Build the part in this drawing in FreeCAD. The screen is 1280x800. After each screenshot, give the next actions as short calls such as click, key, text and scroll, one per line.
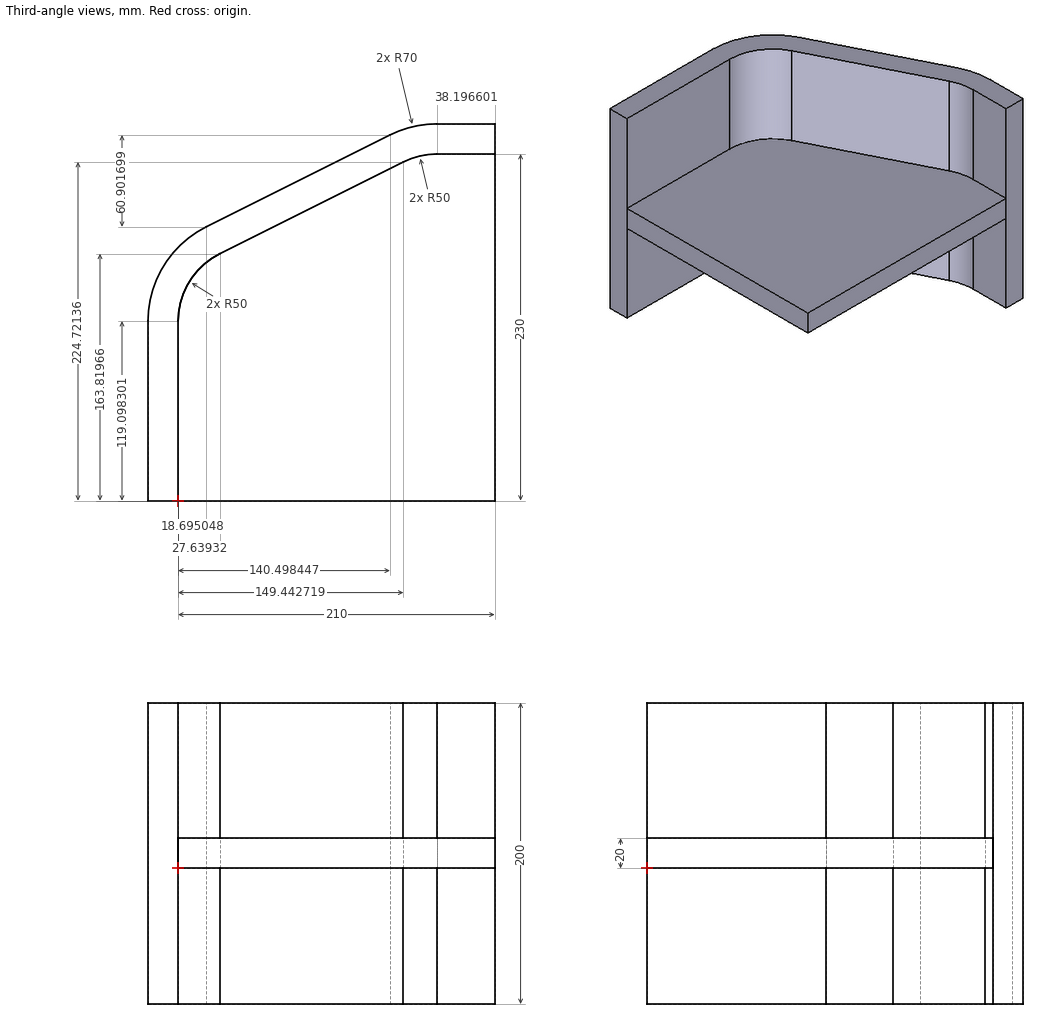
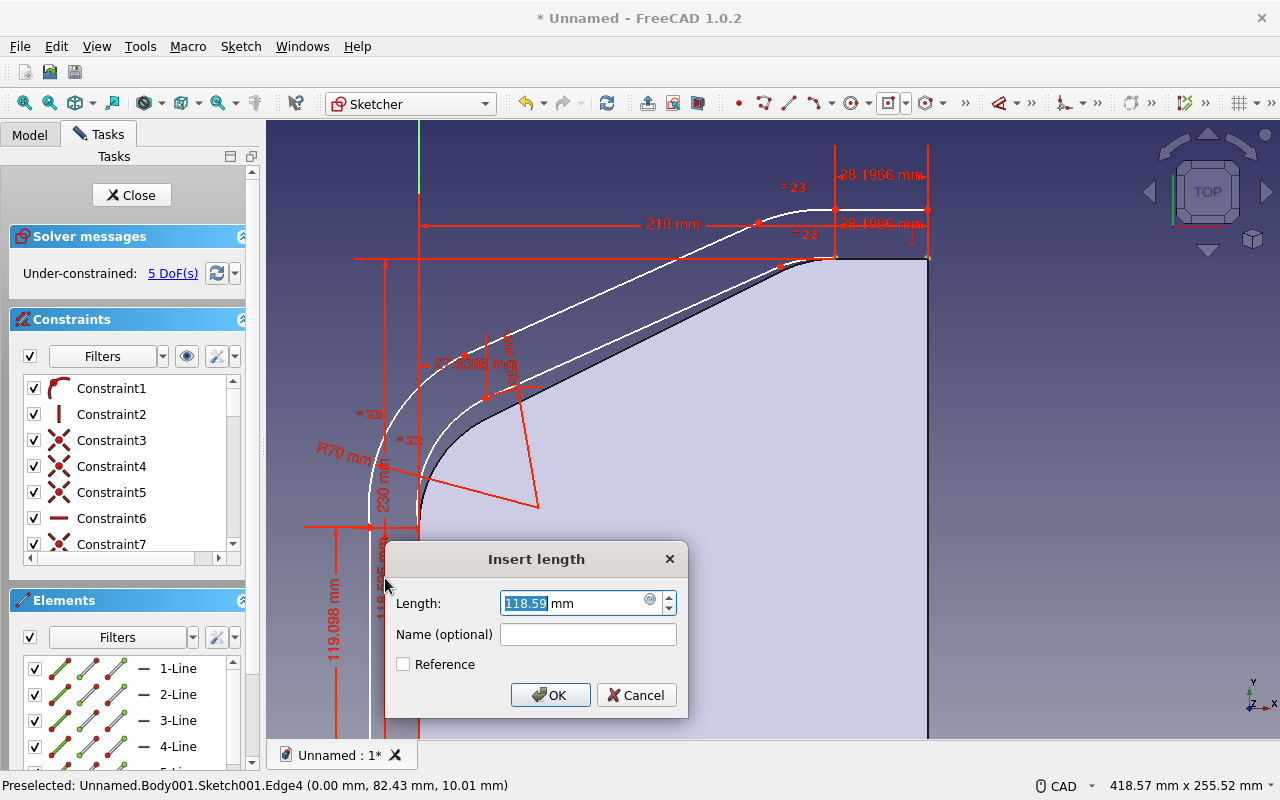
text(119.098301)
key(Return)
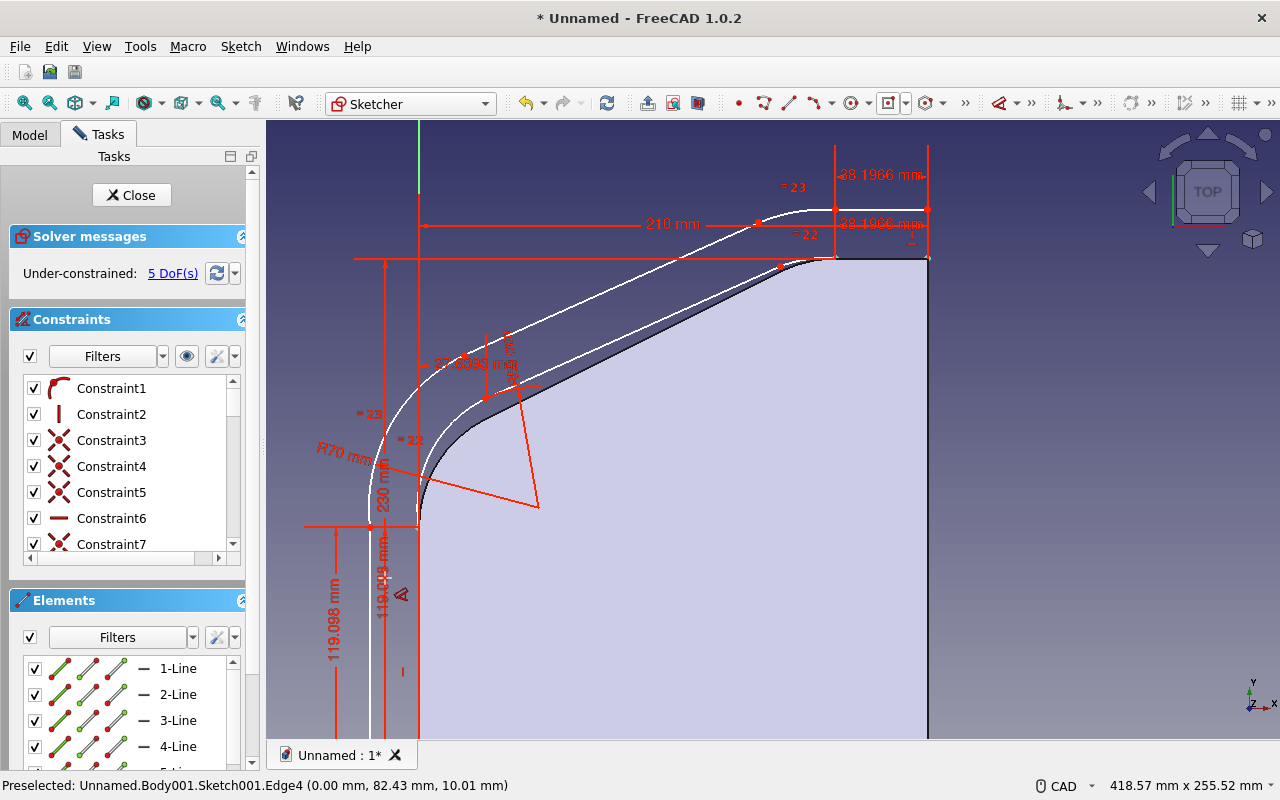
click(465, 355)
click(442, 321)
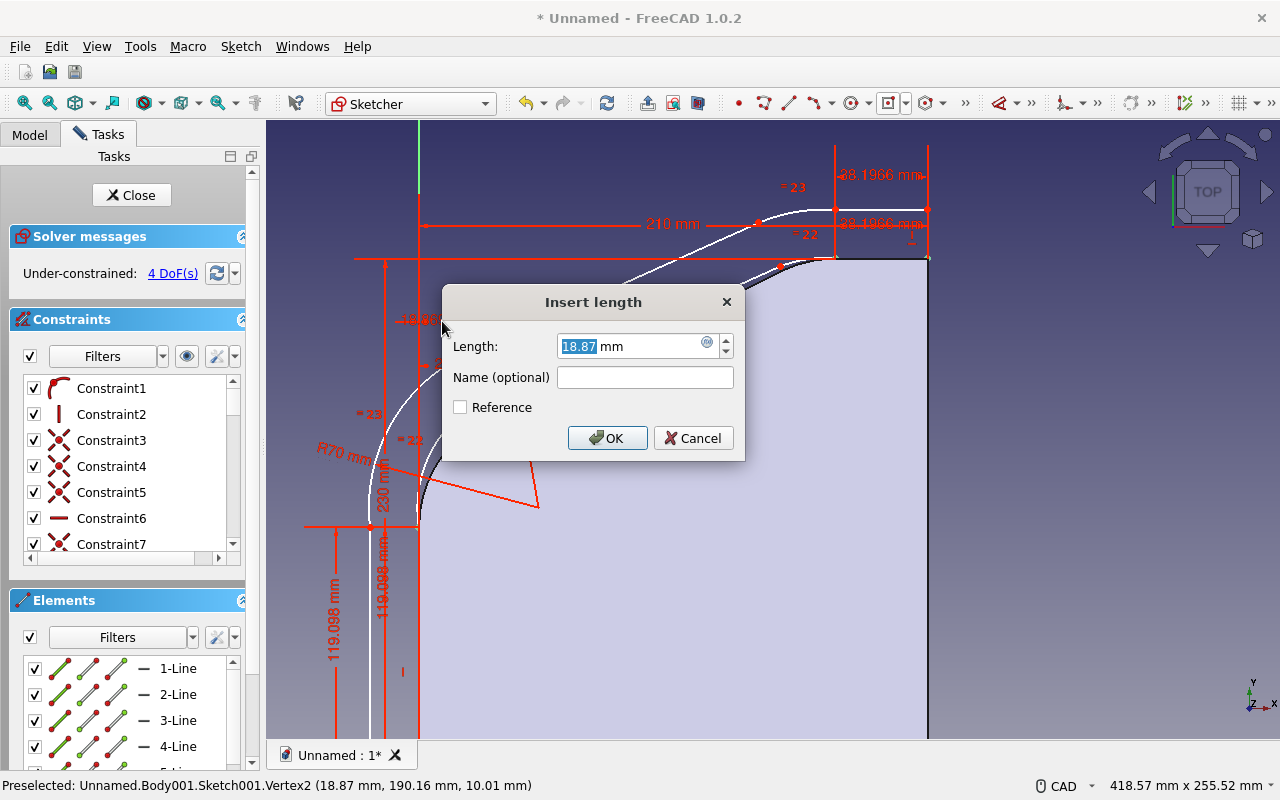
text(18.695048)
key(Return)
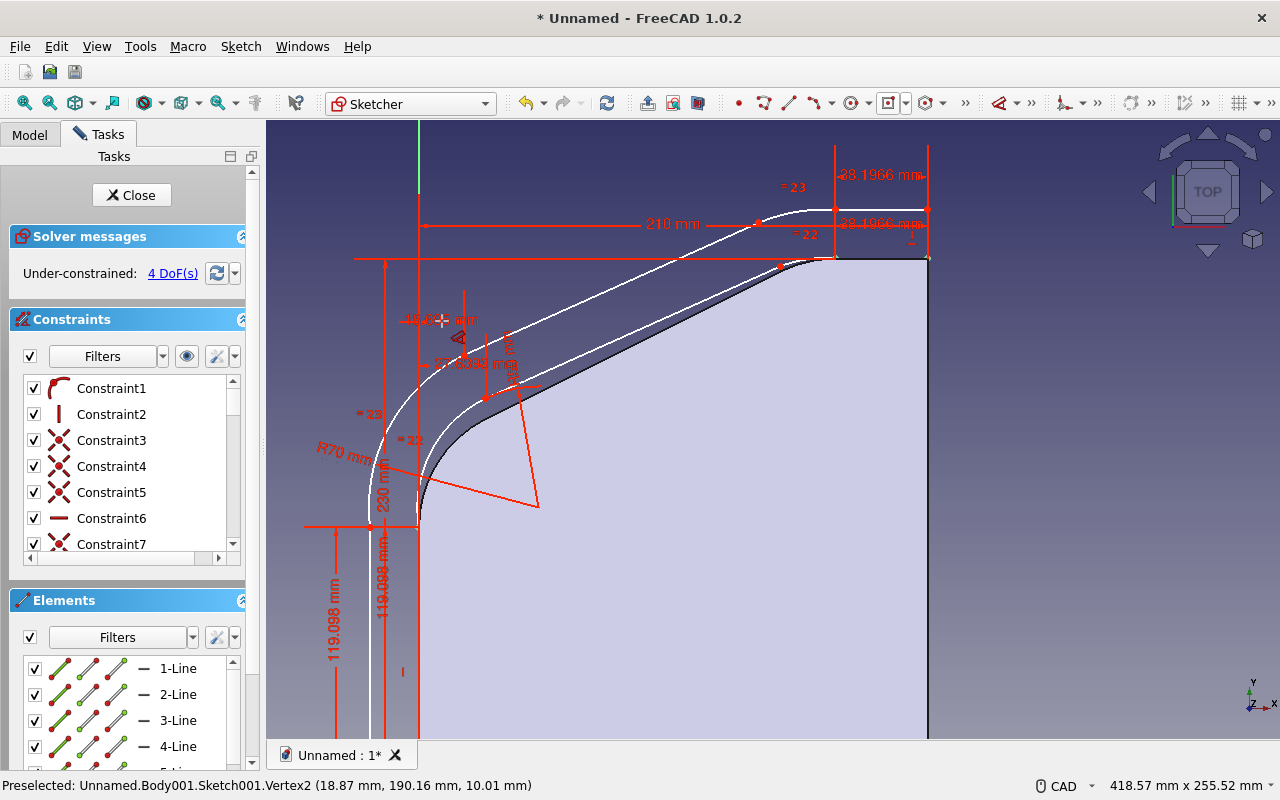
click(486, 398)
click(385, 555)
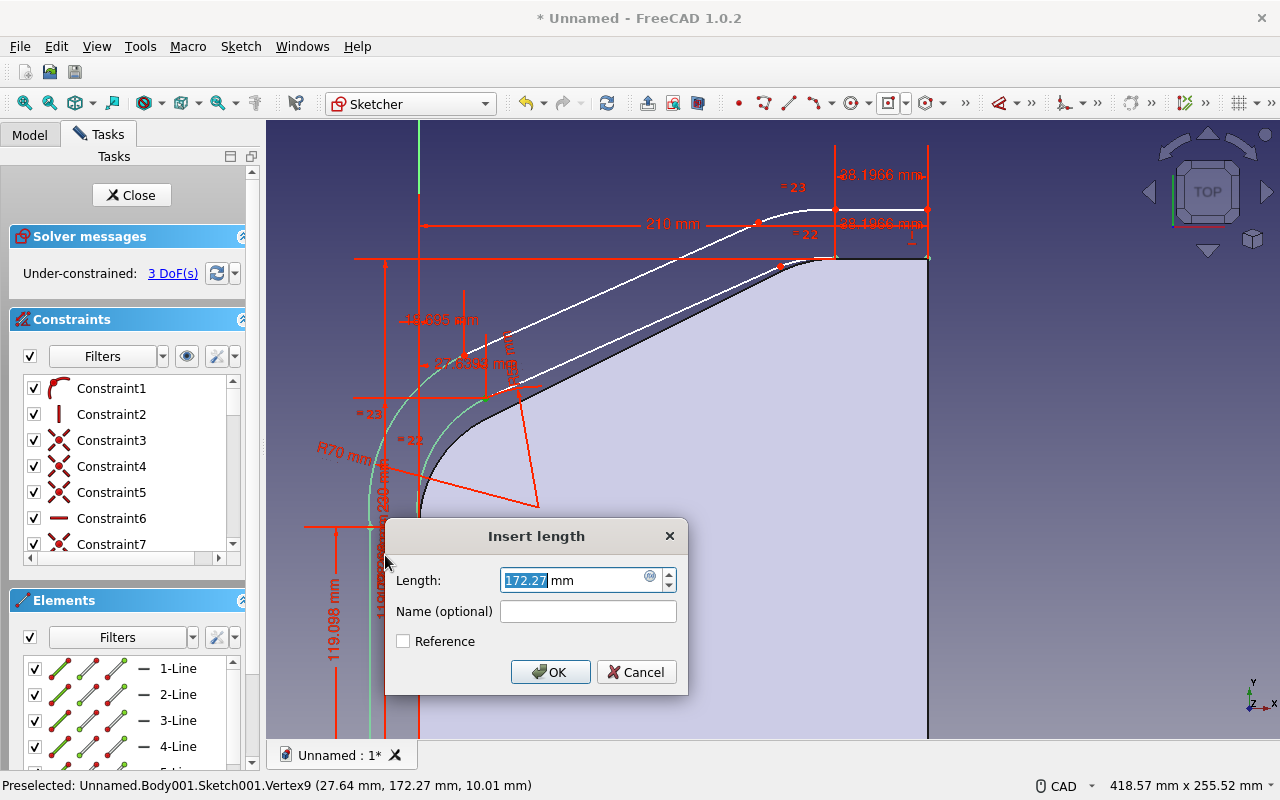
text(163.81966)
key(Return)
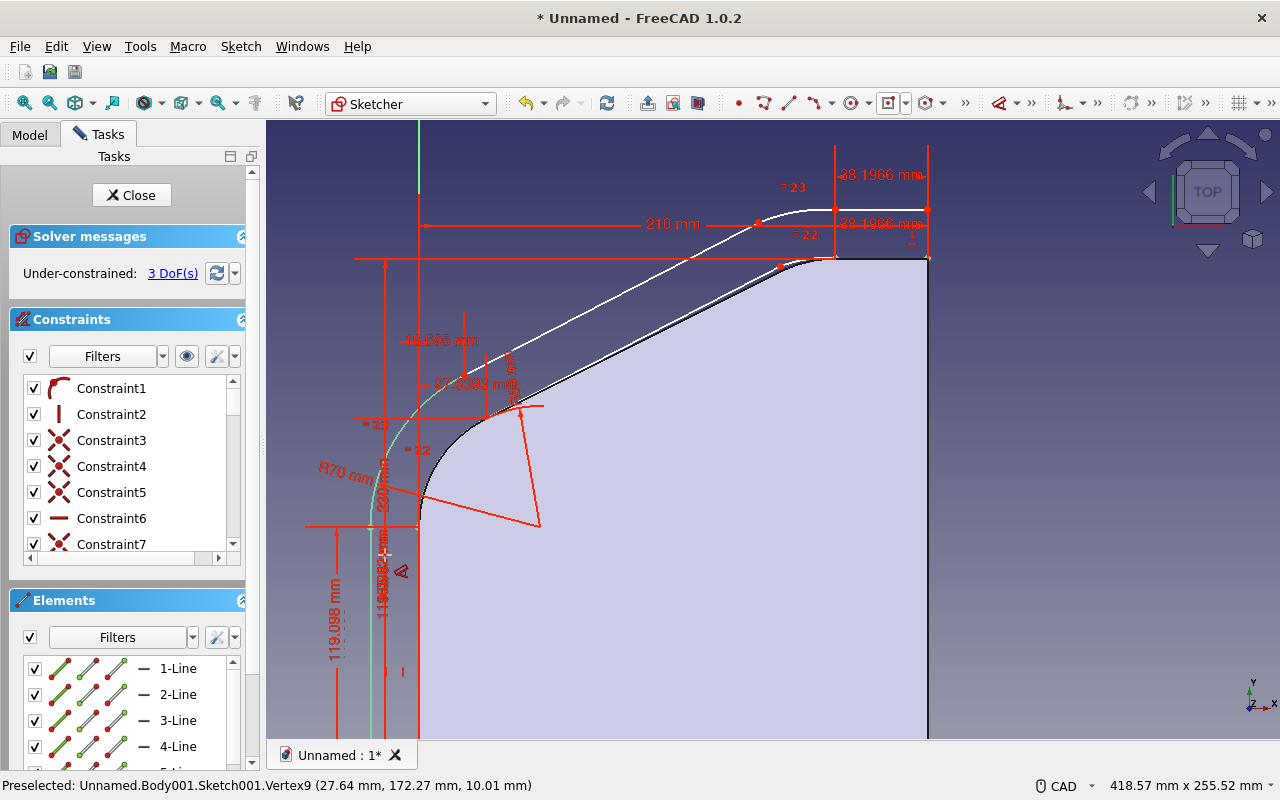
click(781, 266)
click(385, 386)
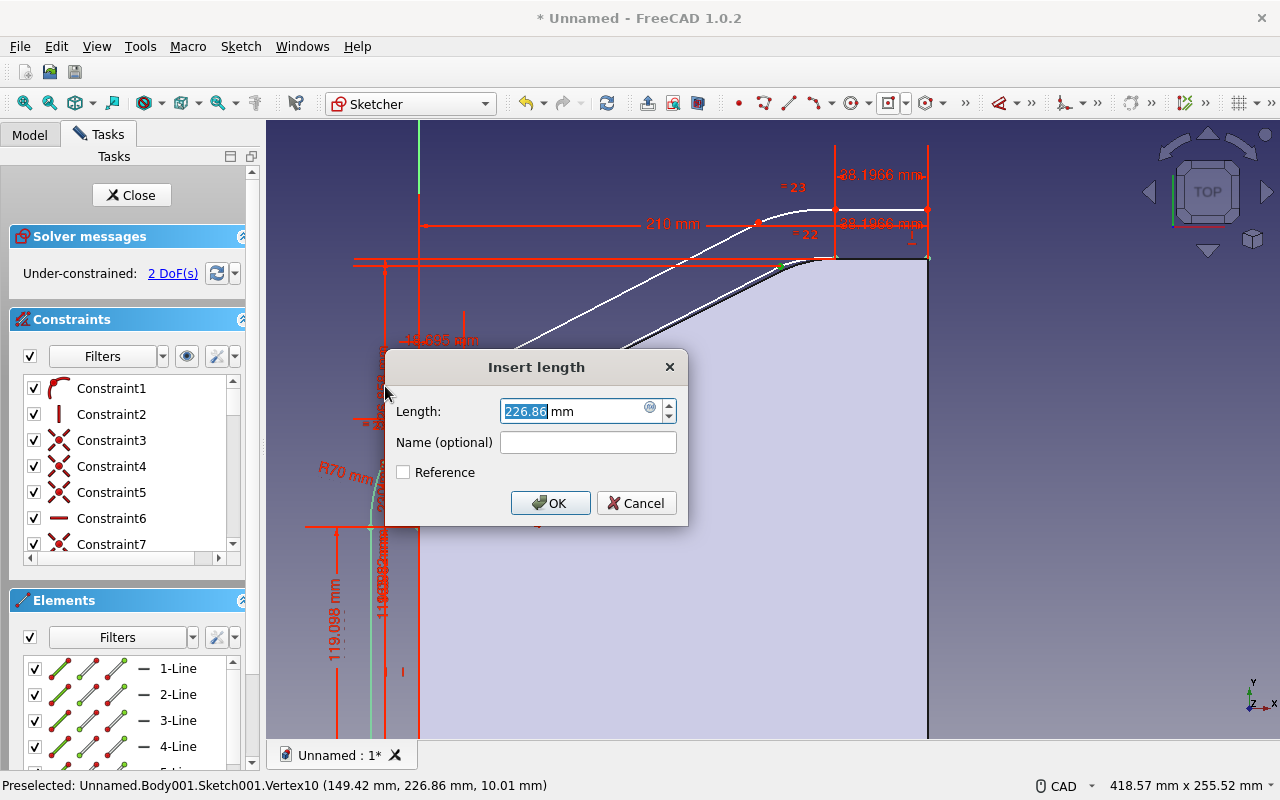
text(224.72136)
key(Return)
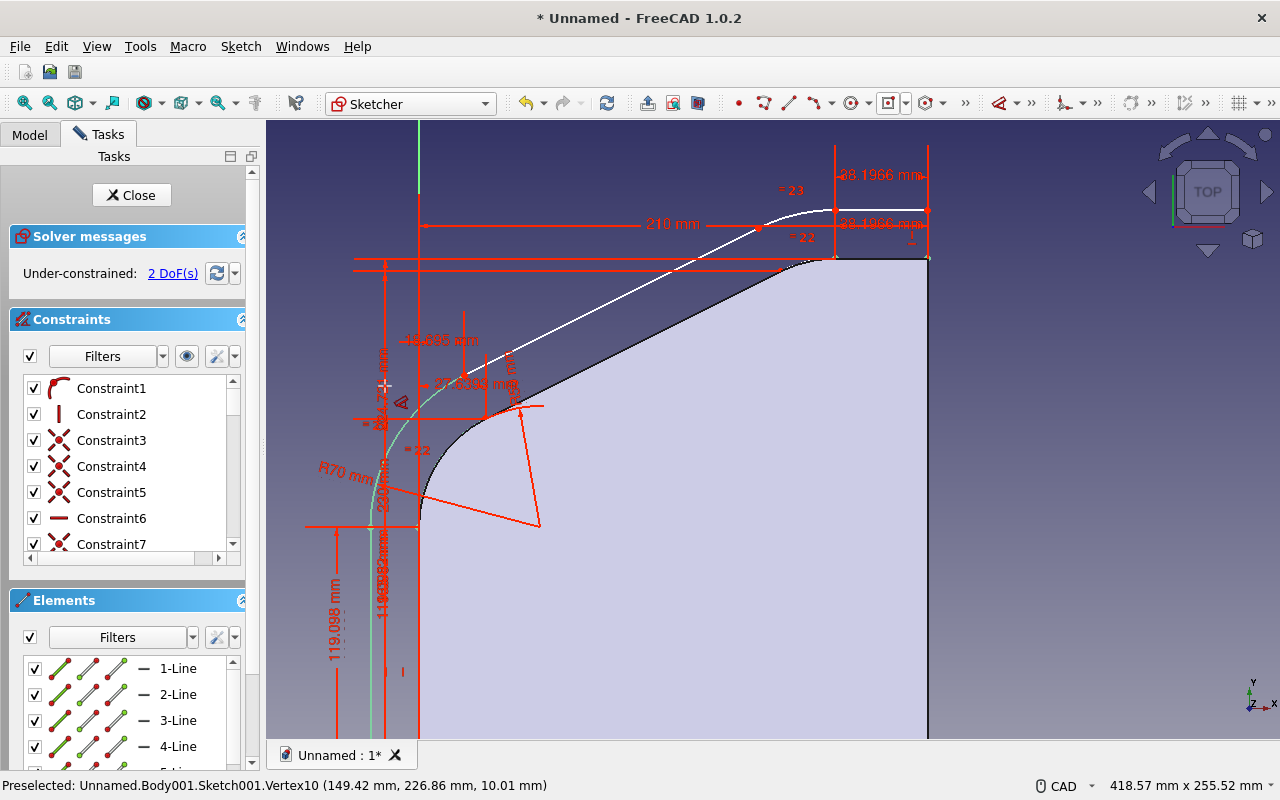
click(670, 272)
click(793, 302)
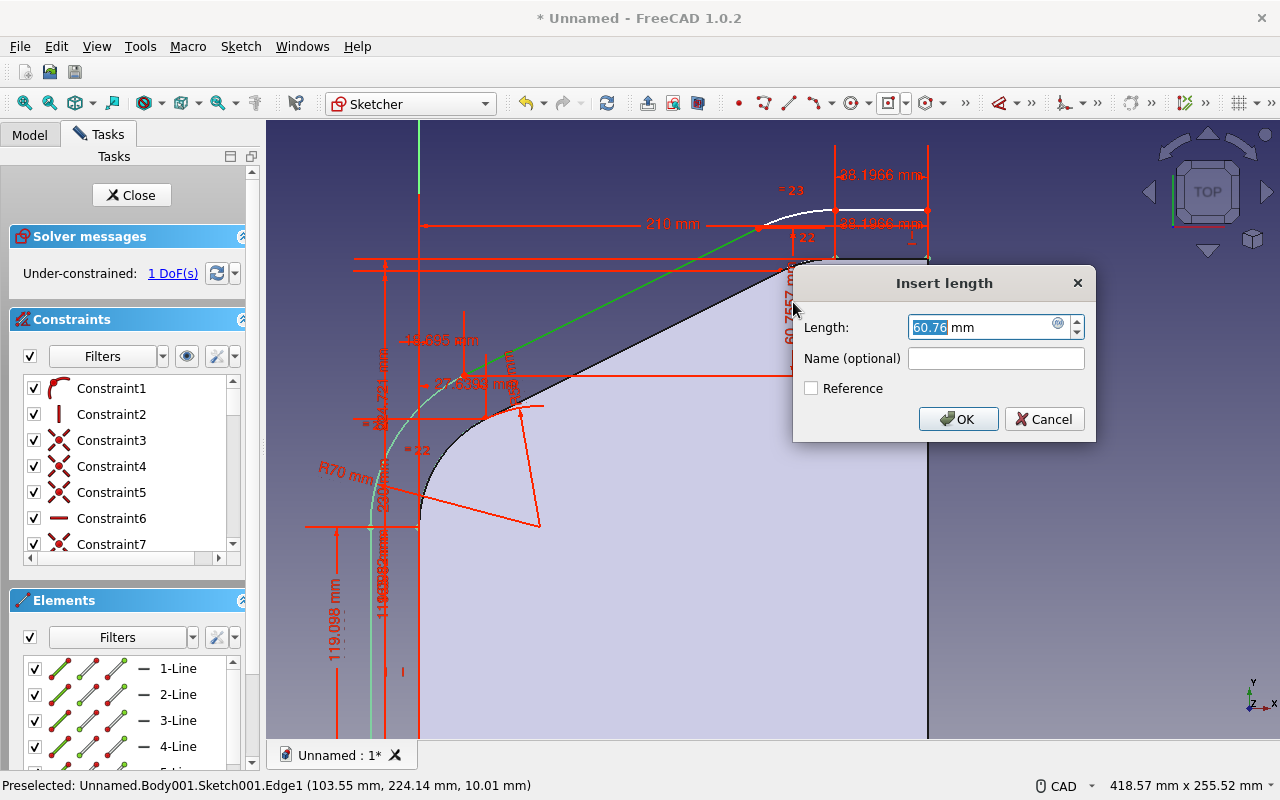
text(60.901699)
key(Return)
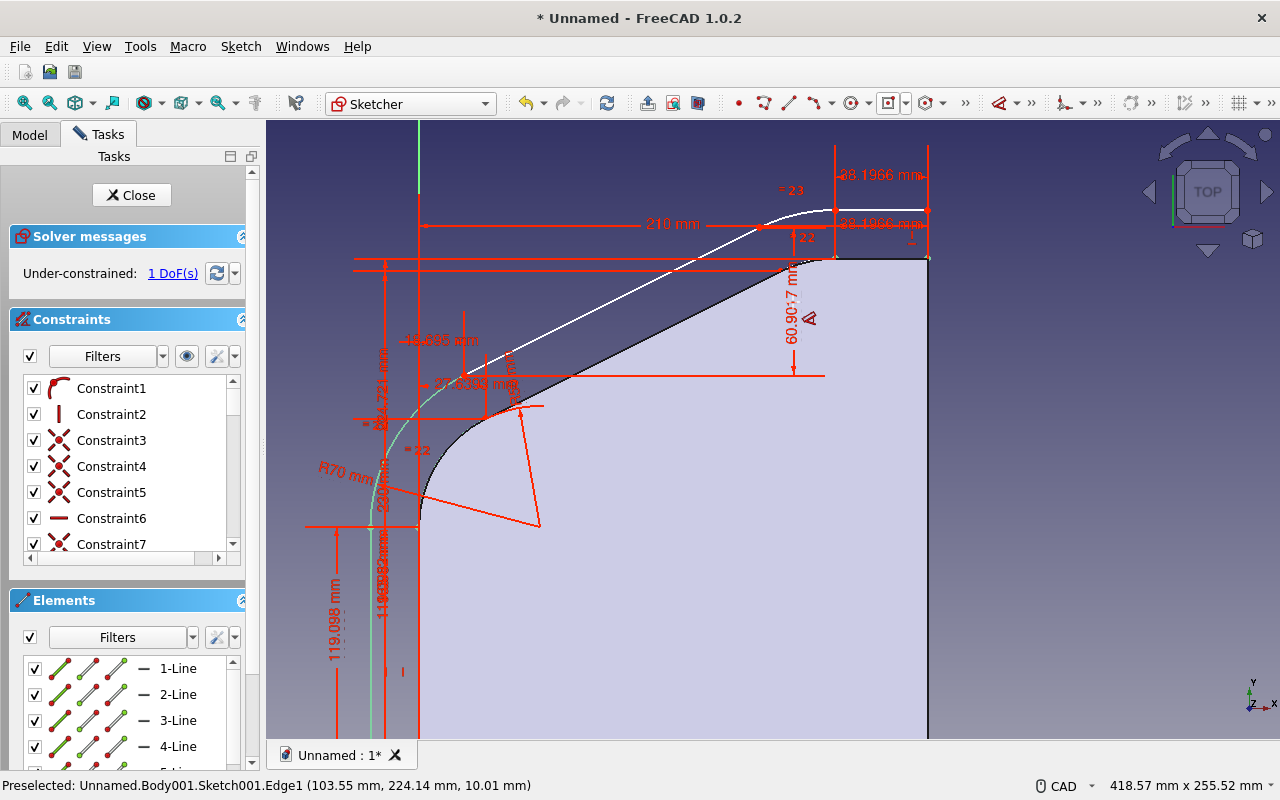
click(759, 228)
click(589, 194)